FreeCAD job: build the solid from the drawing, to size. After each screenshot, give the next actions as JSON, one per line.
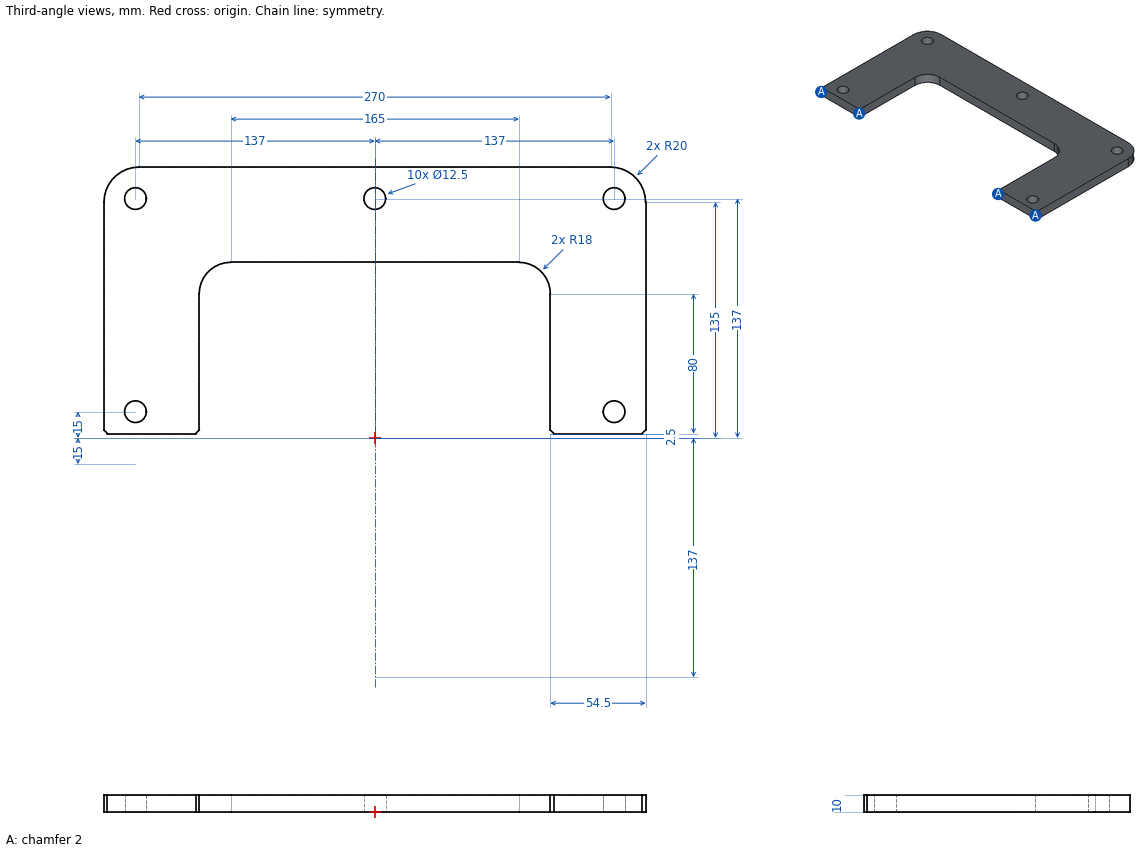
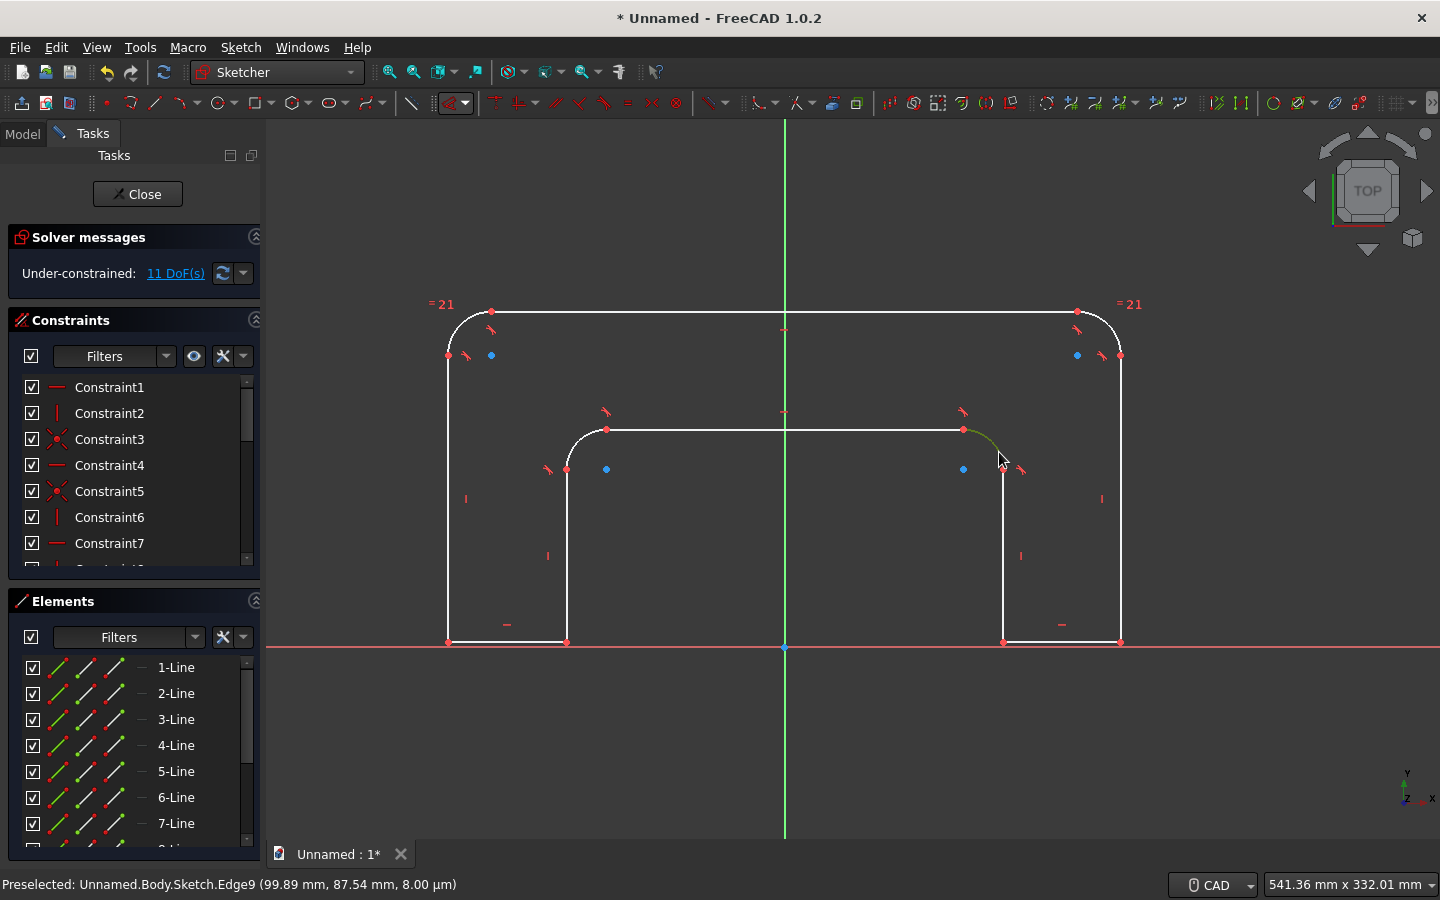
{"action": "left_click", "coordinate": [588, 434]}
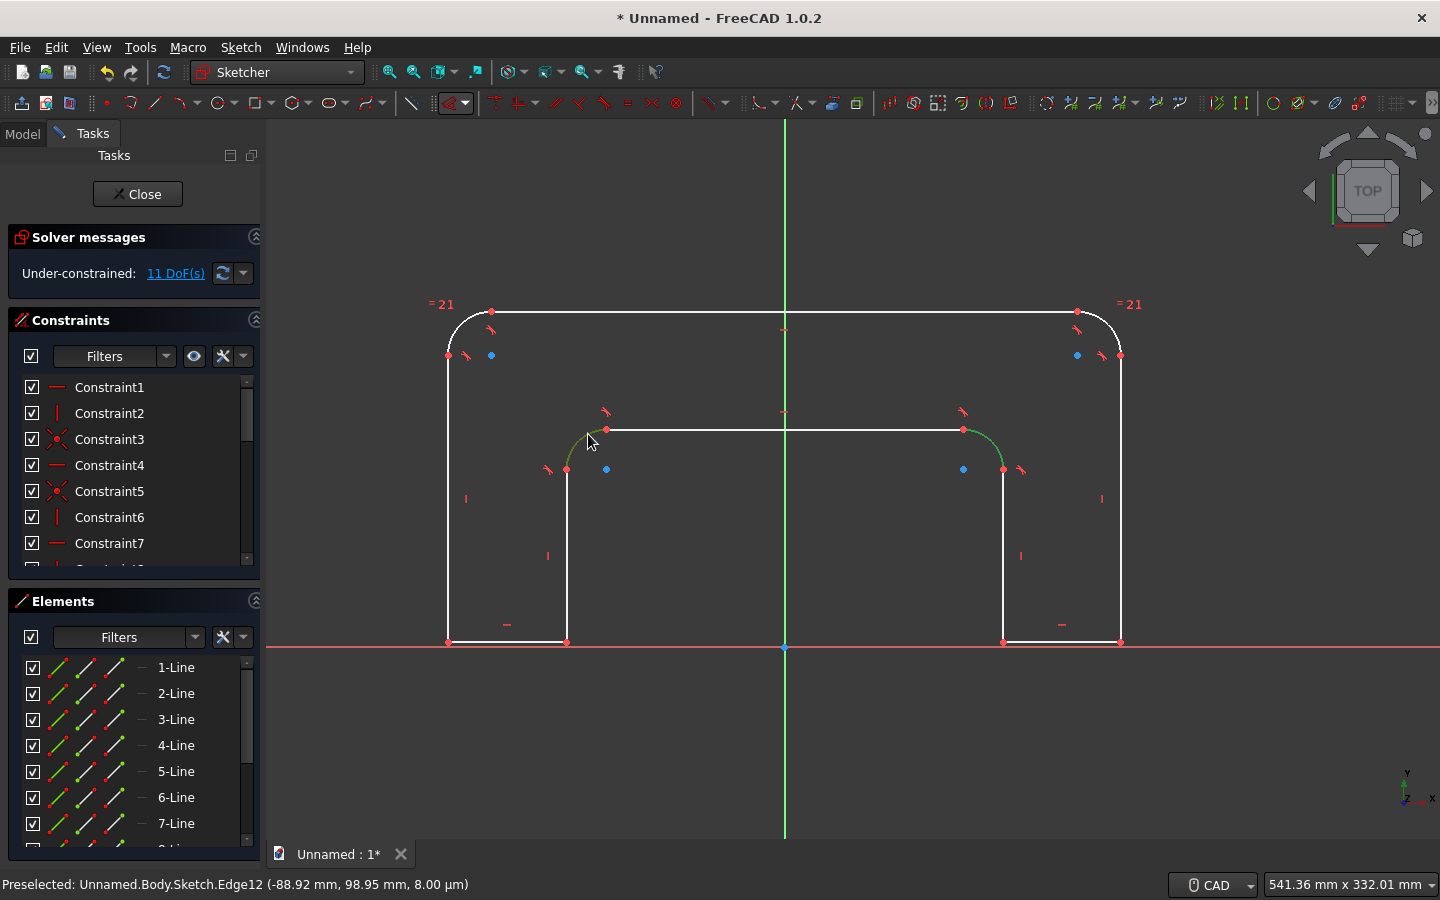
{"action": "key", "text": "e"}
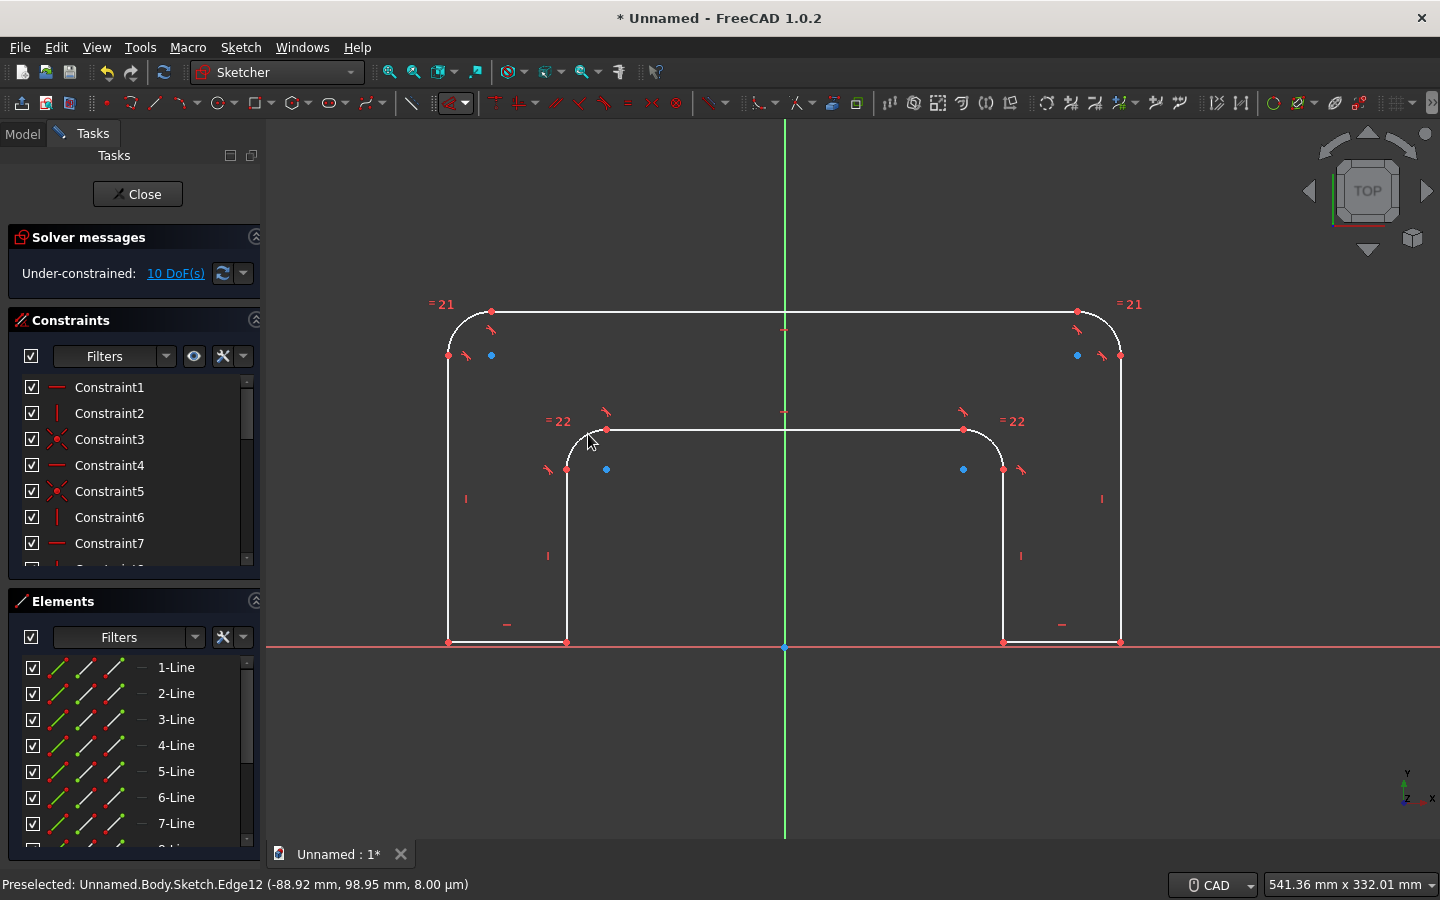
{"action": "left_click", "coordinate": [1121, 642]}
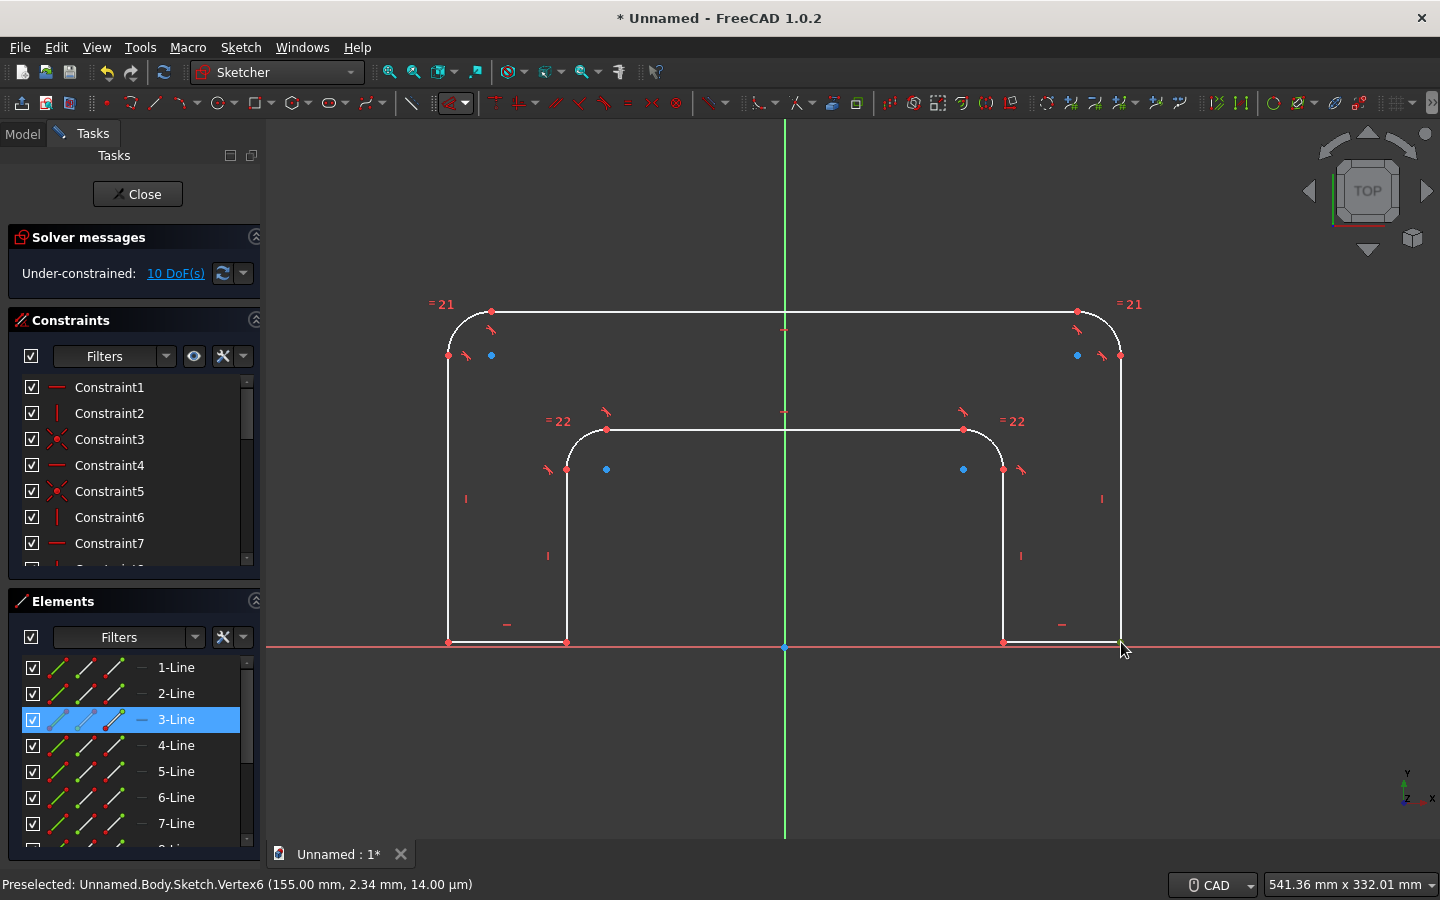
{"action": "left_click", "coordinate": [448, 642]}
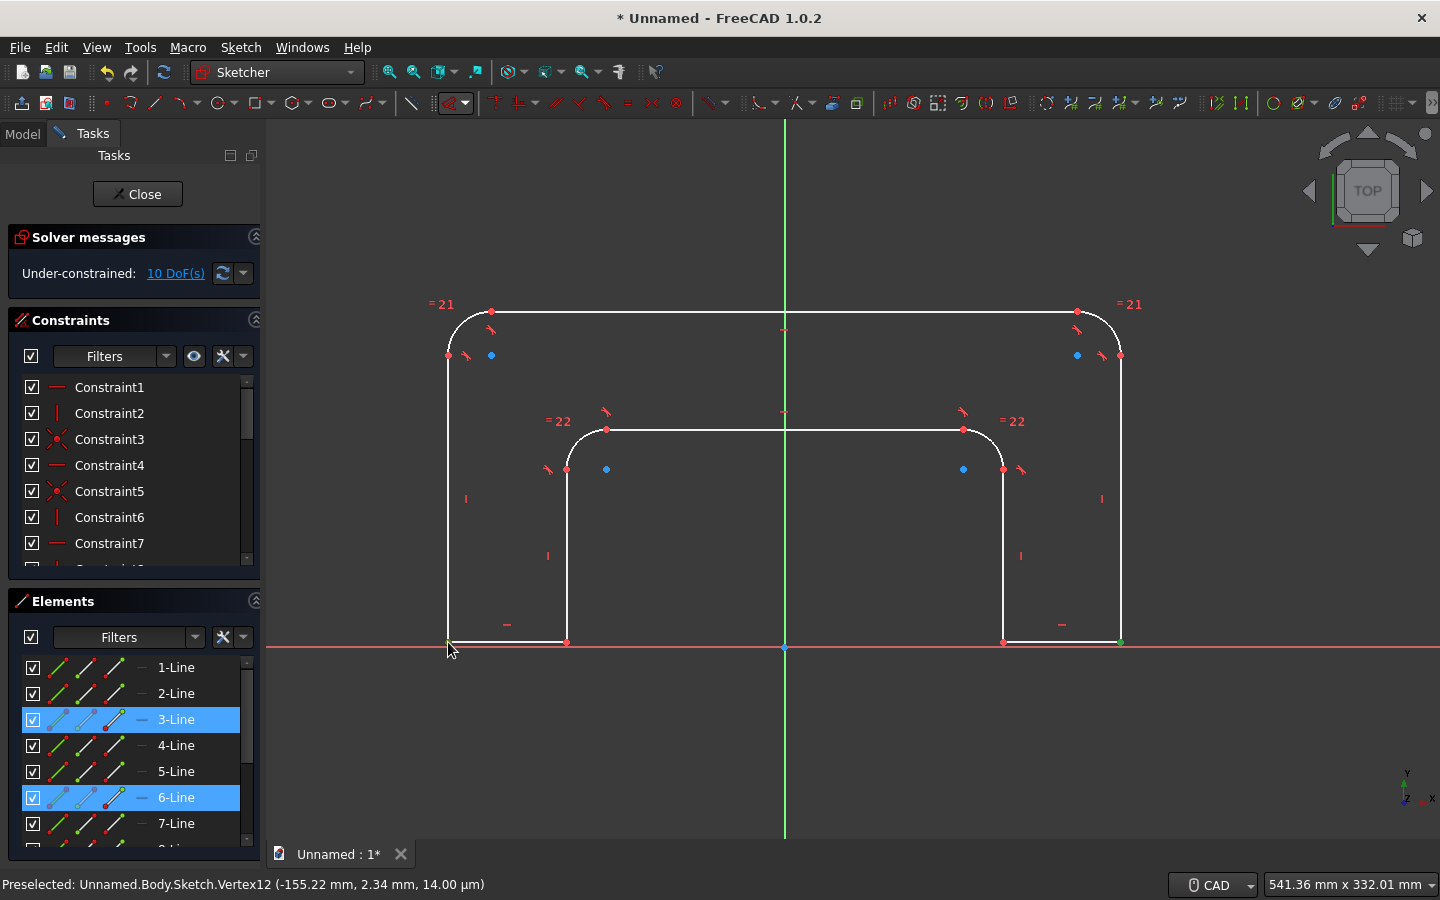
{"action": "left_click", "coordinate": [785, 764]}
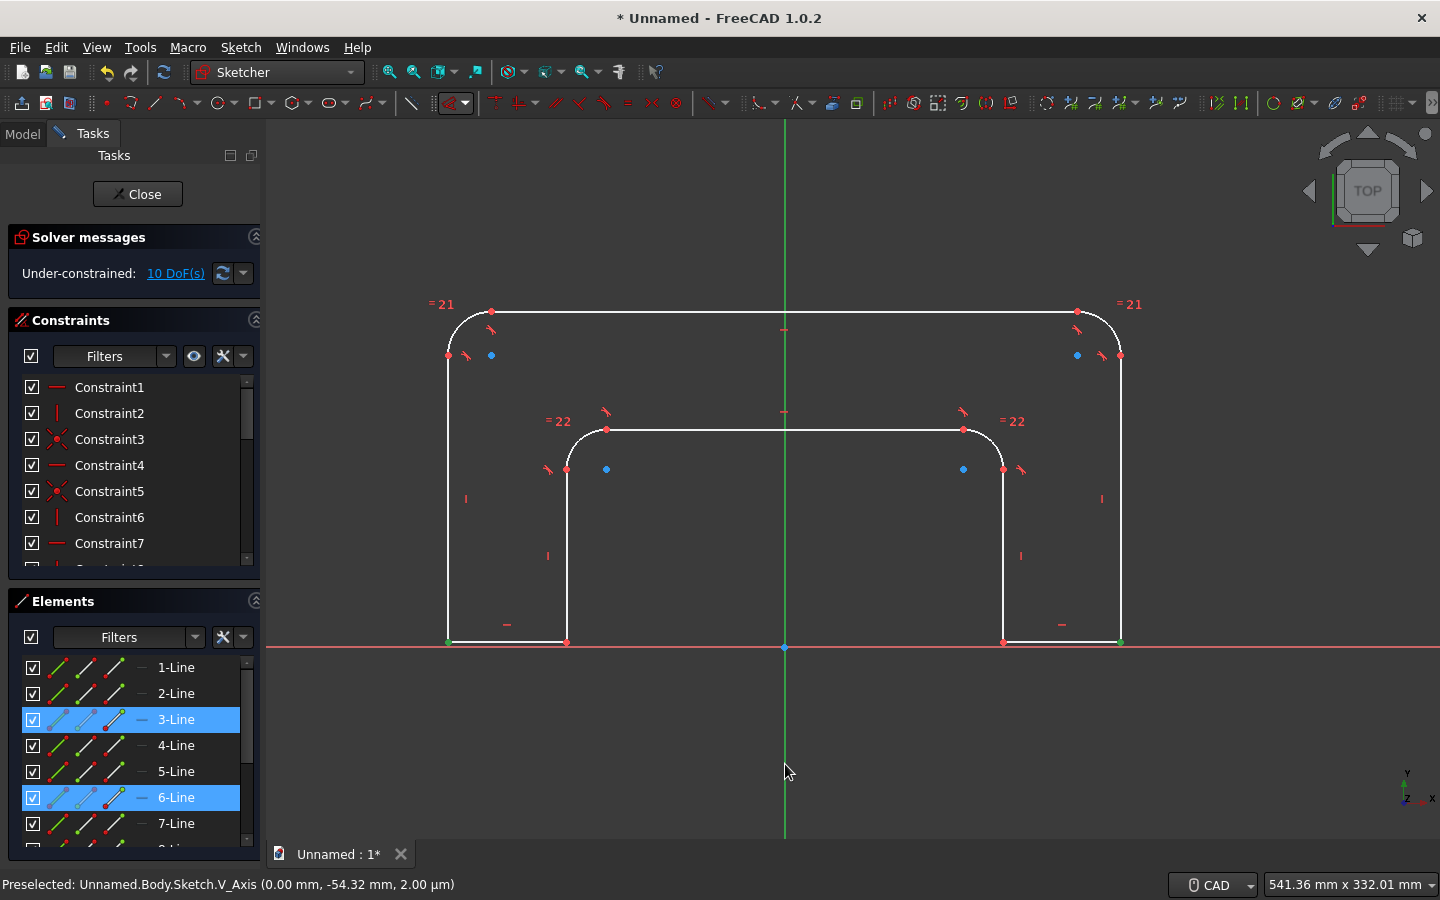
{"action": "key", "text": "s"}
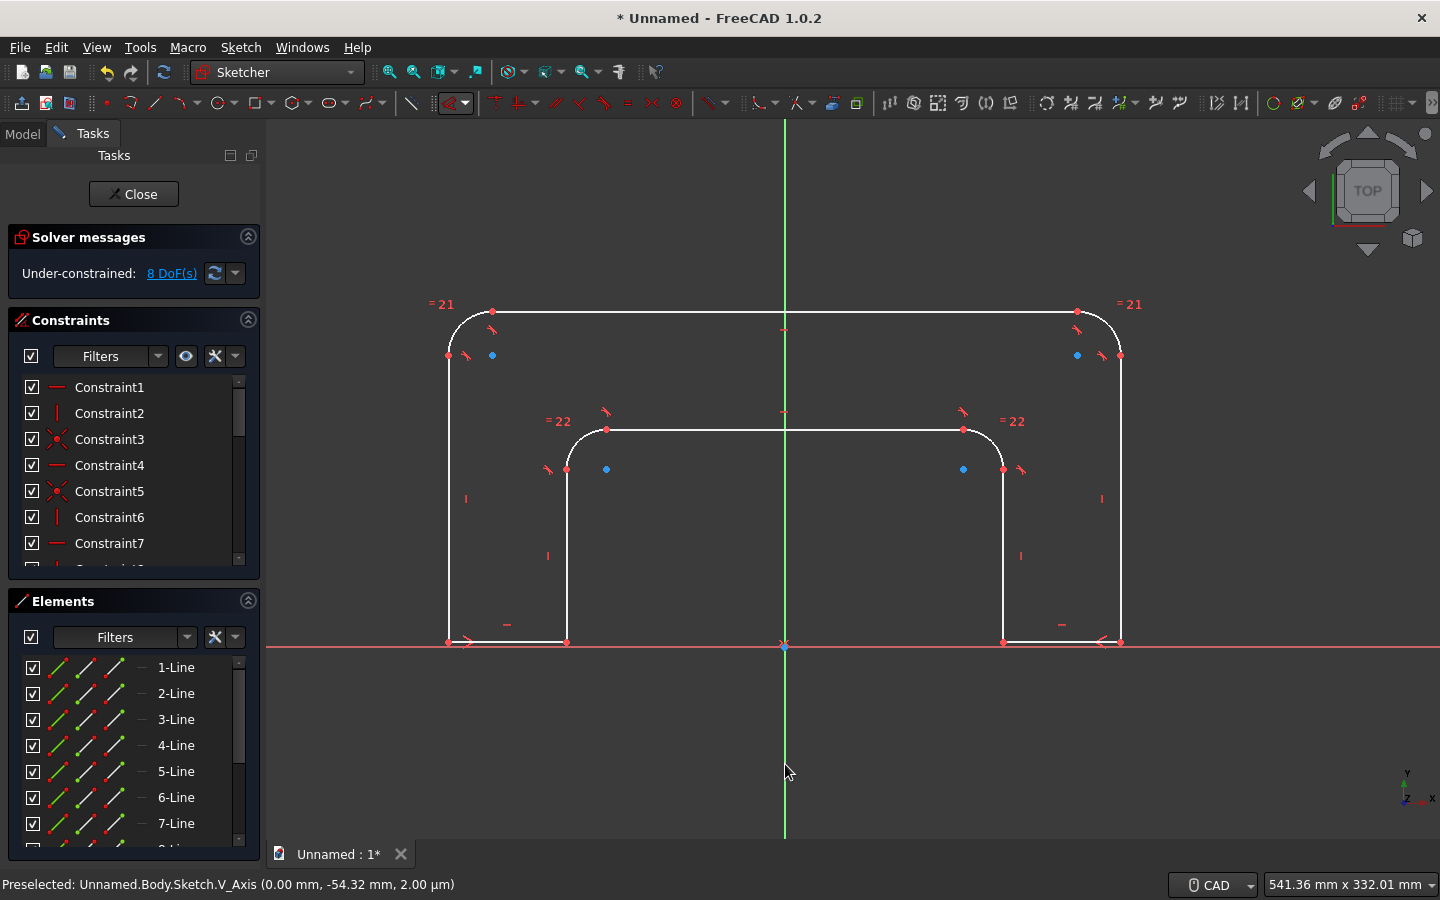
{"action": "left_click", "coordinate": [999, 452]}